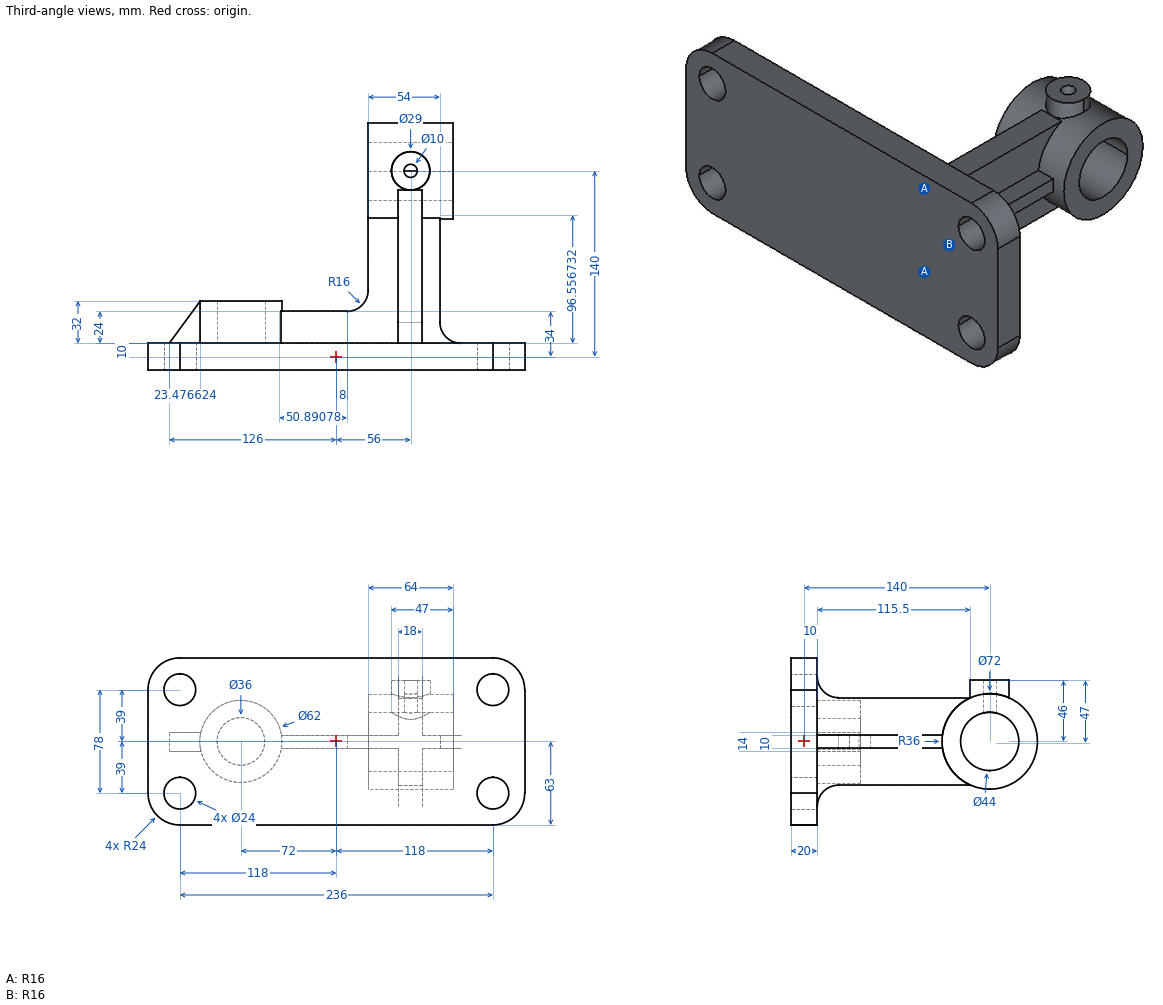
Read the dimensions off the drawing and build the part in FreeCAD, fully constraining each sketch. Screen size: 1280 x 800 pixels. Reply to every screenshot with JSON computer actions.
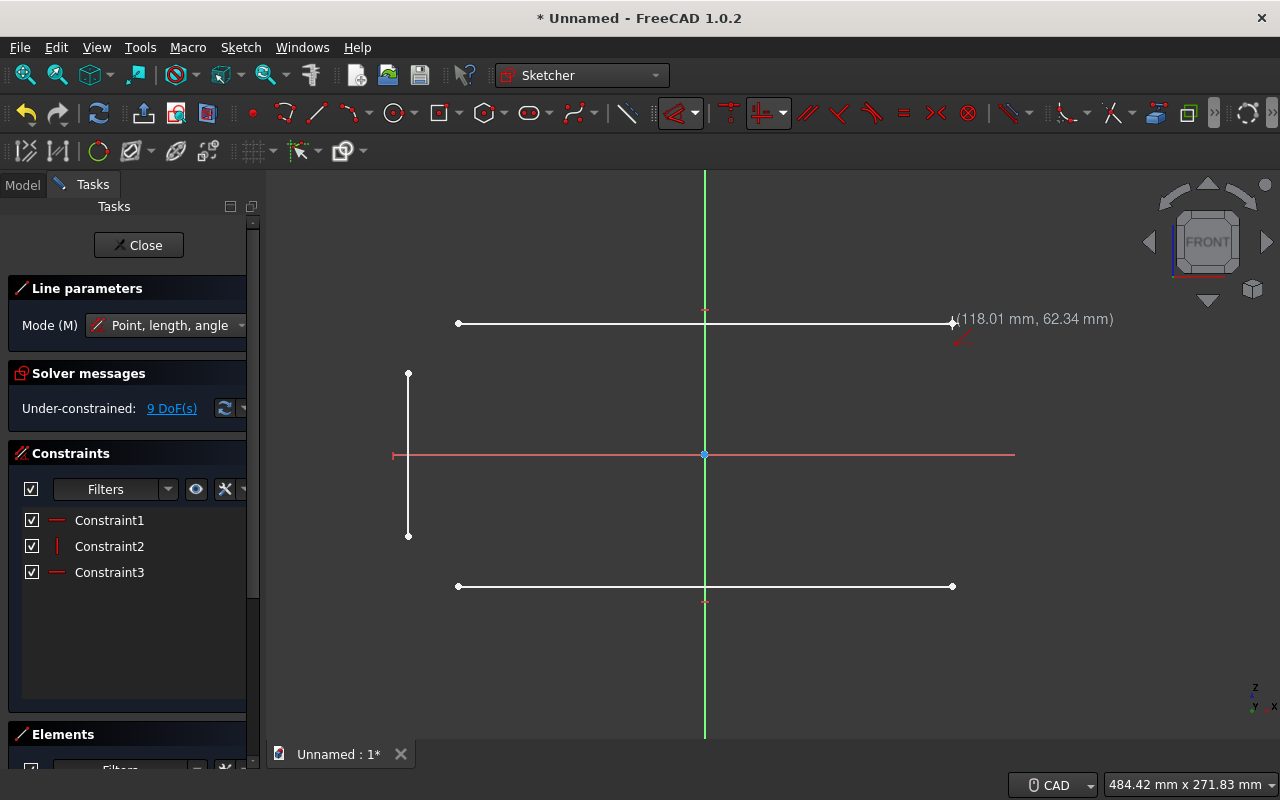
{"action": "left_click", "coordinate": [1002, 373]}
{"action": "left_click", "coordinate": [1002, 536]}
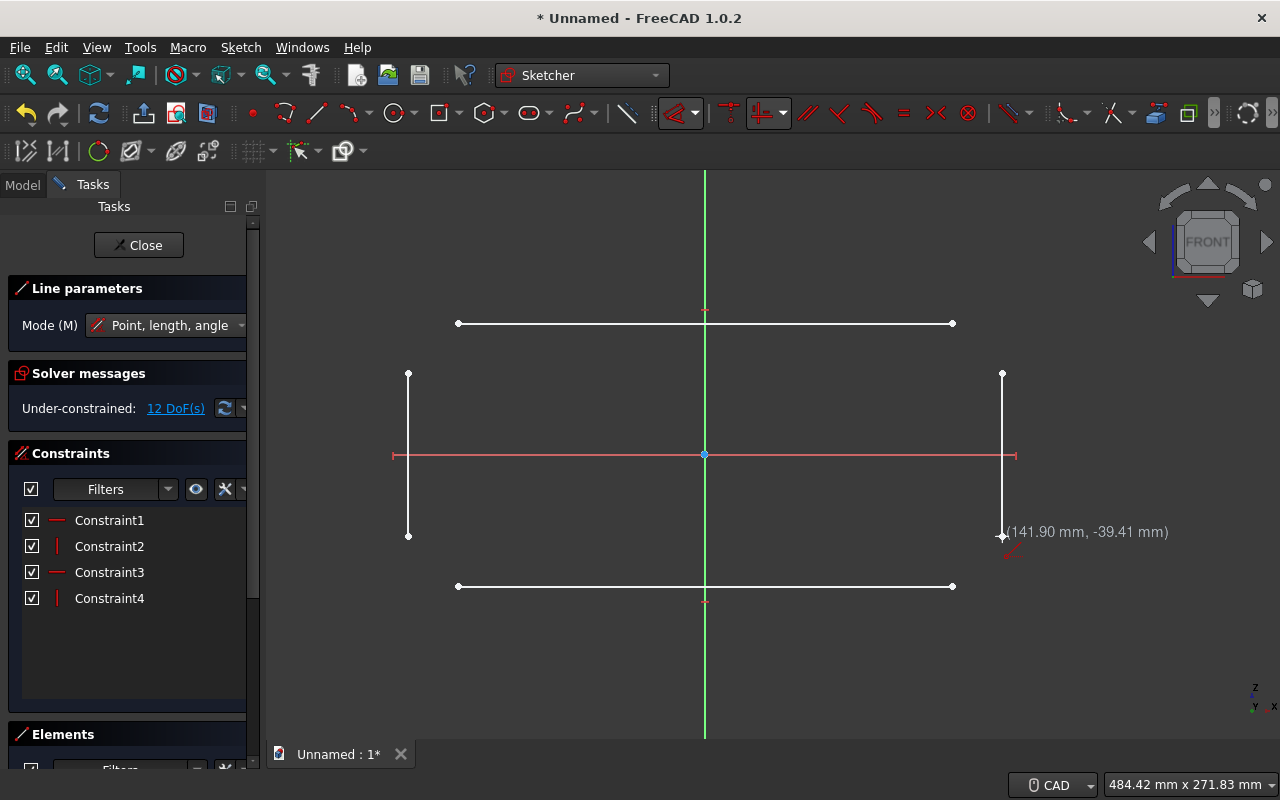
{"action": "left_click", "coordinate": [350, 114]}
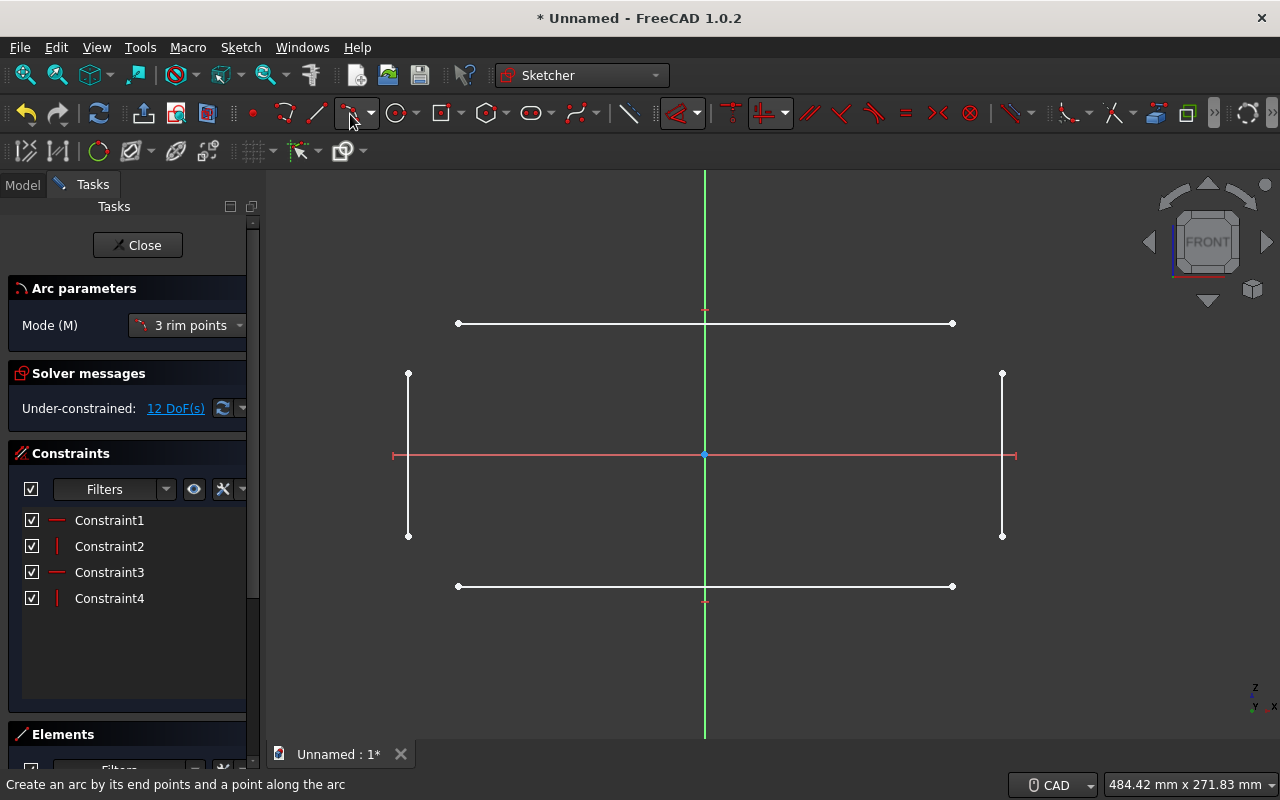
{"action": "left_click", "coordinate": [458, 587]}
{"action": "left_click", "coordinate": [408, 537]}
{"action": "left_click", "coordinate": [422, 572]}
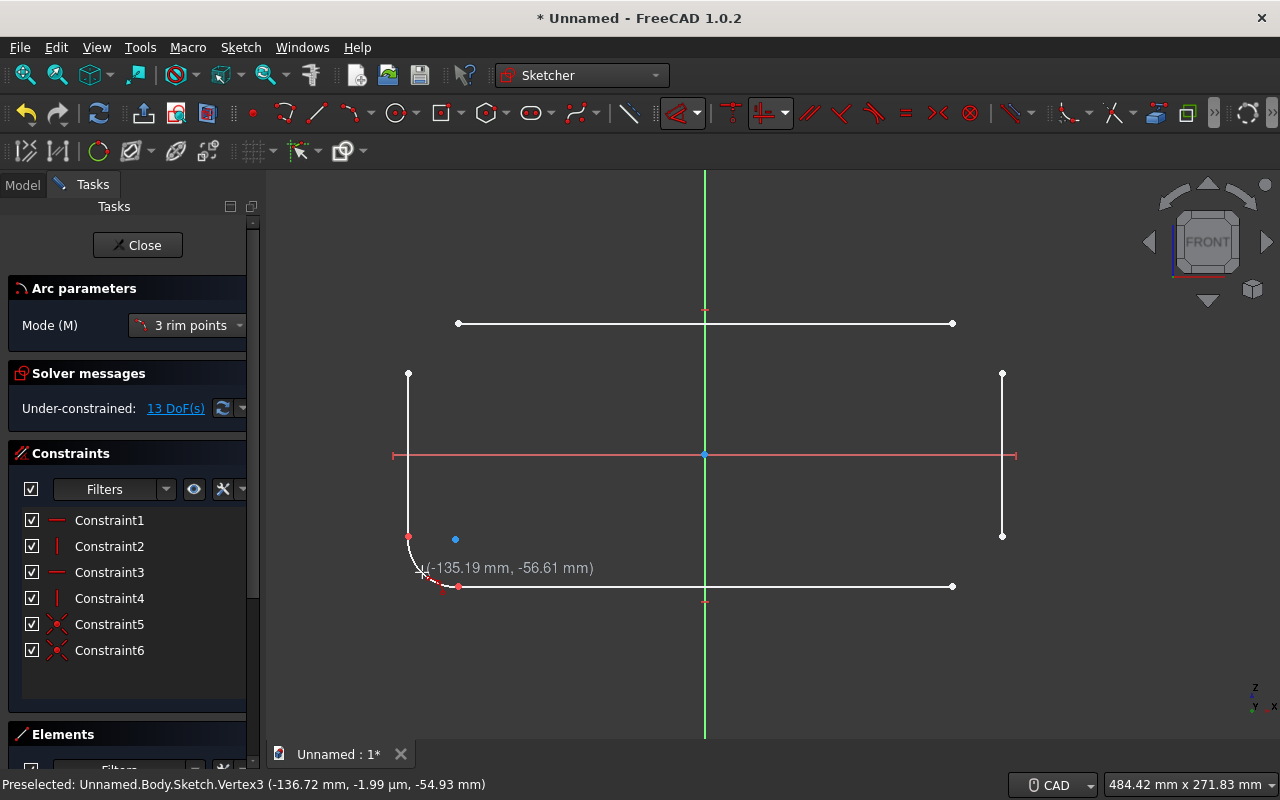
{"action": "left_click", "coordinate": [408, 374]}
{"action": "left_click", "coordinate": [458, 324]}
{"action": "left_click", "coordinate": [422, 337]}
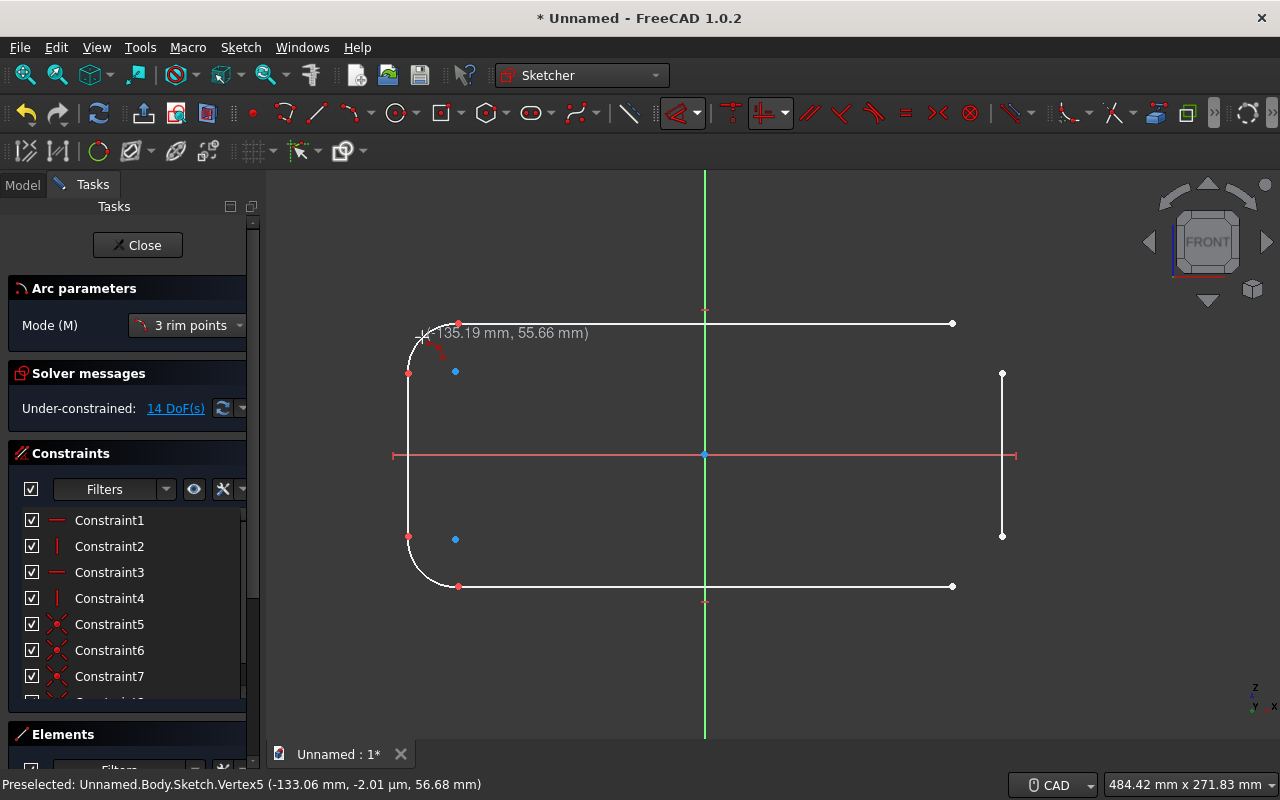
{"action": "left_click", "coordinate": [952, 324]}
{"action": "left_click", "coordinate": [1002, 374]}
{"action": "left_click", "coordinate": [988, 337]}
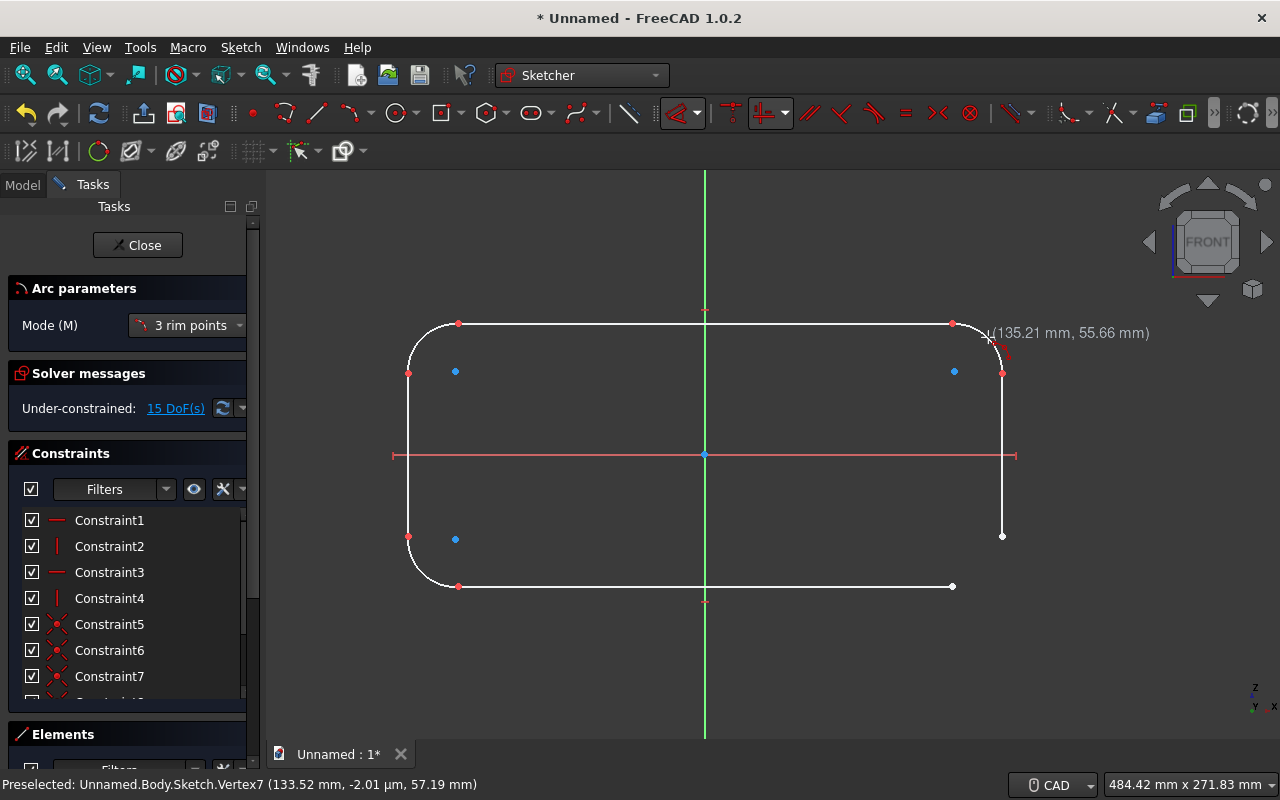
{"action": "left_click", "coordinate": [1002, 537]}
{"action": "left_click", "coordinate": [952, 587]}
{"action": "left_click", "coordinate": [988, 572]}
{"action": "key", "text": "Escape"}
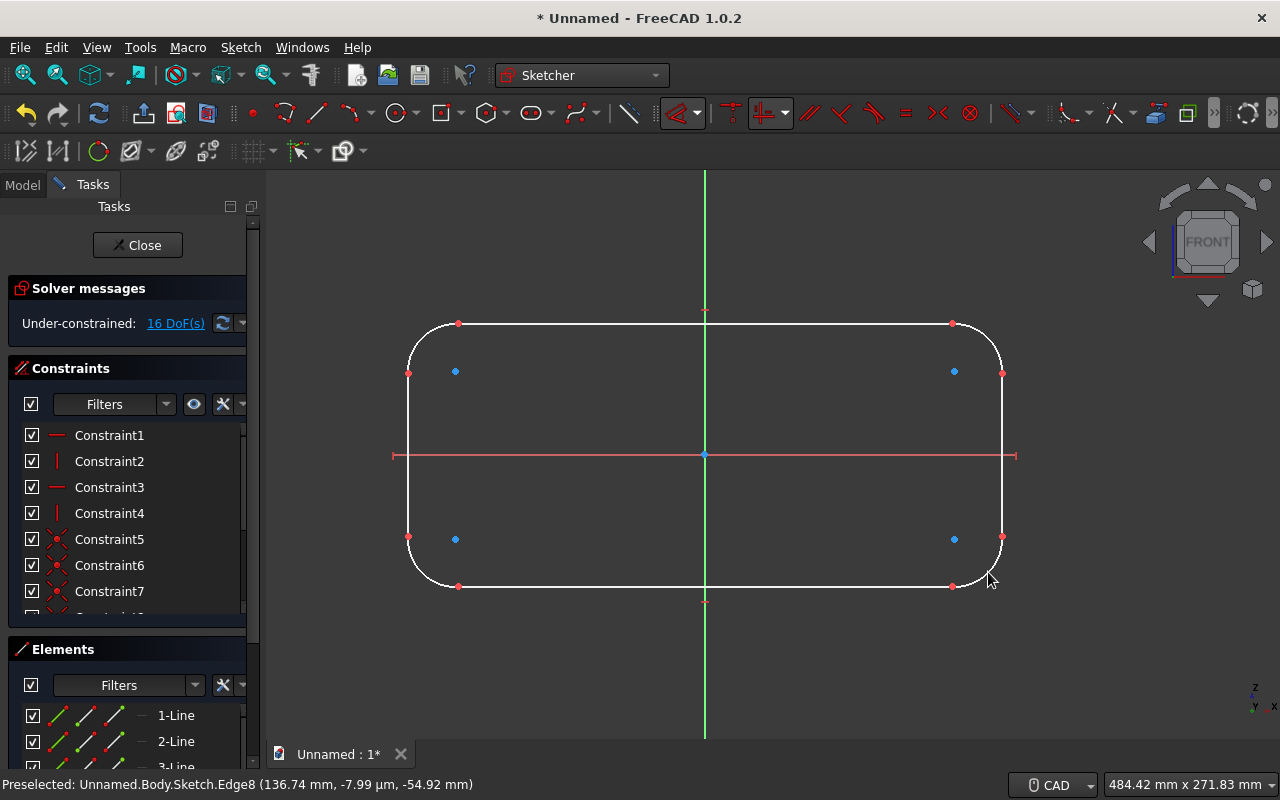
{"action": "left_click", "coordinate": [804, 587]}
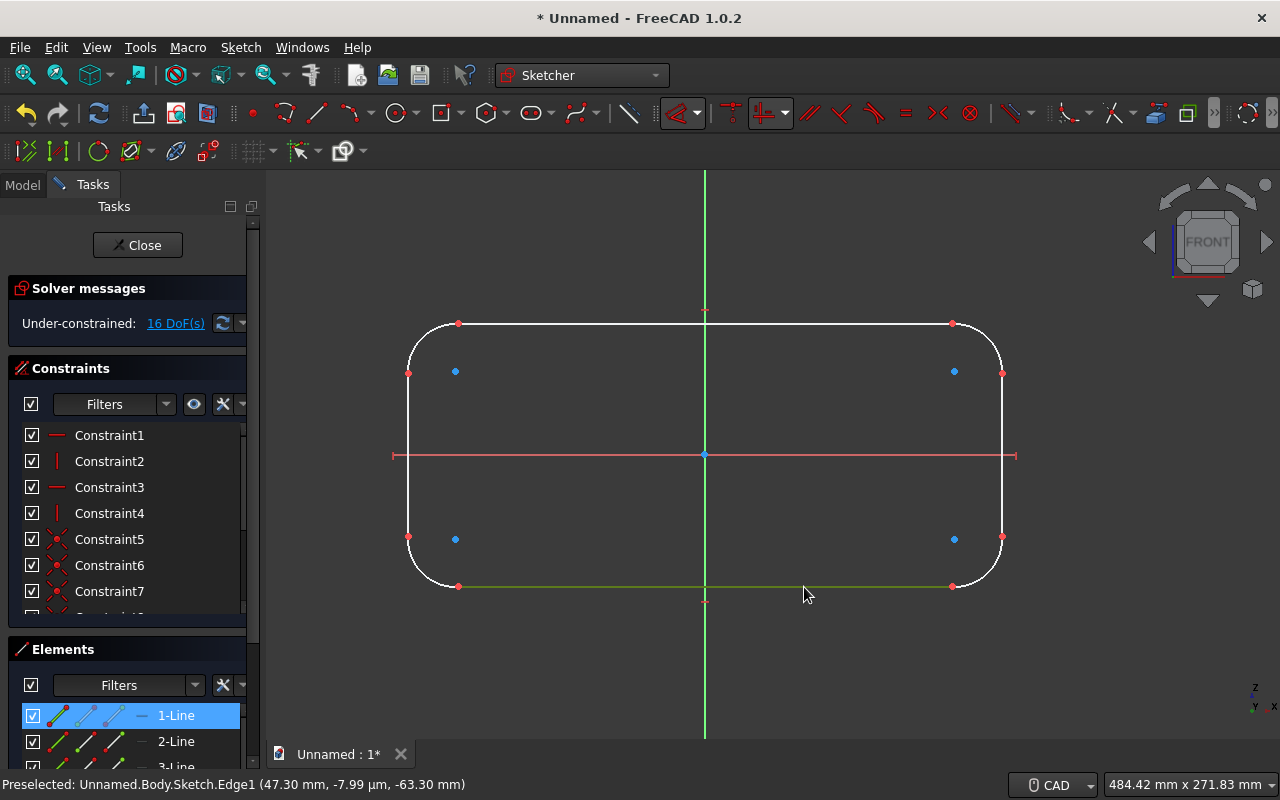
{"action": "left_click", "coordinate": [413, 560]}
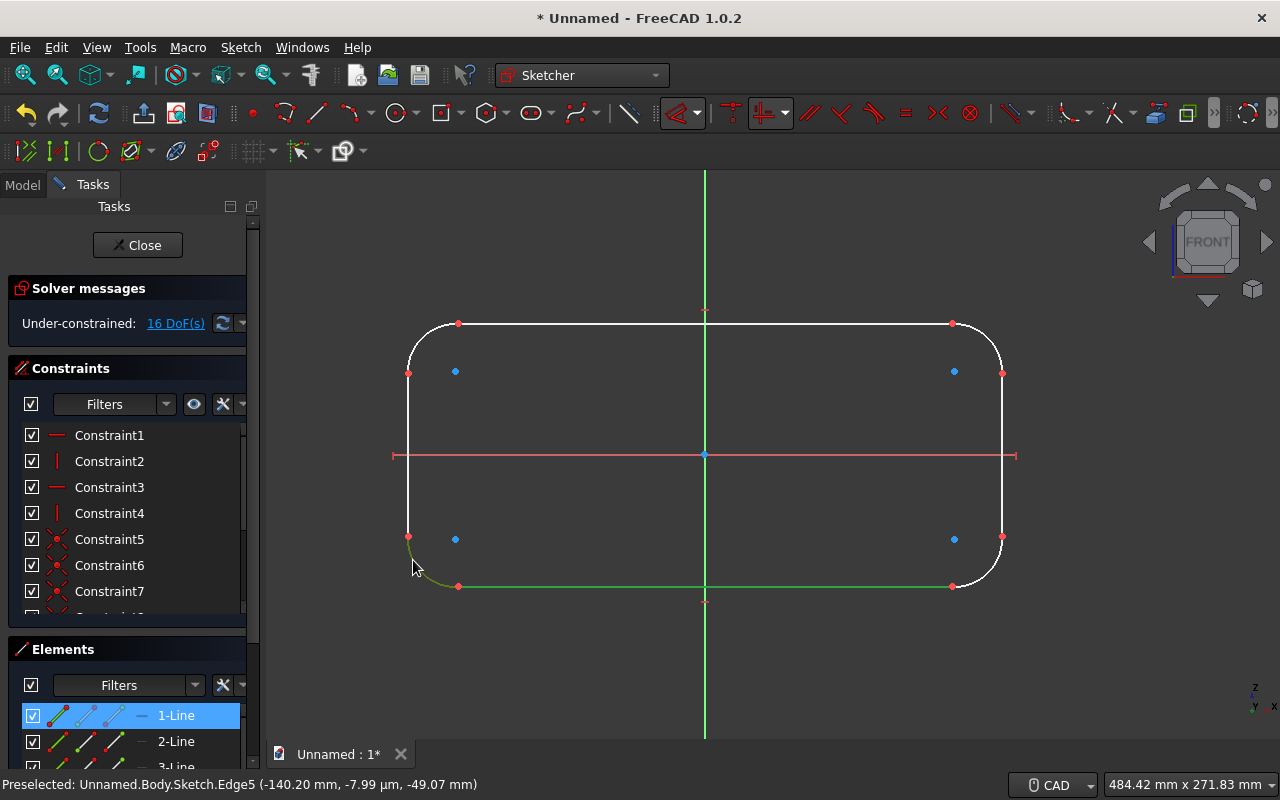
{"action": "left_click", "coordinate": [874, 114]}